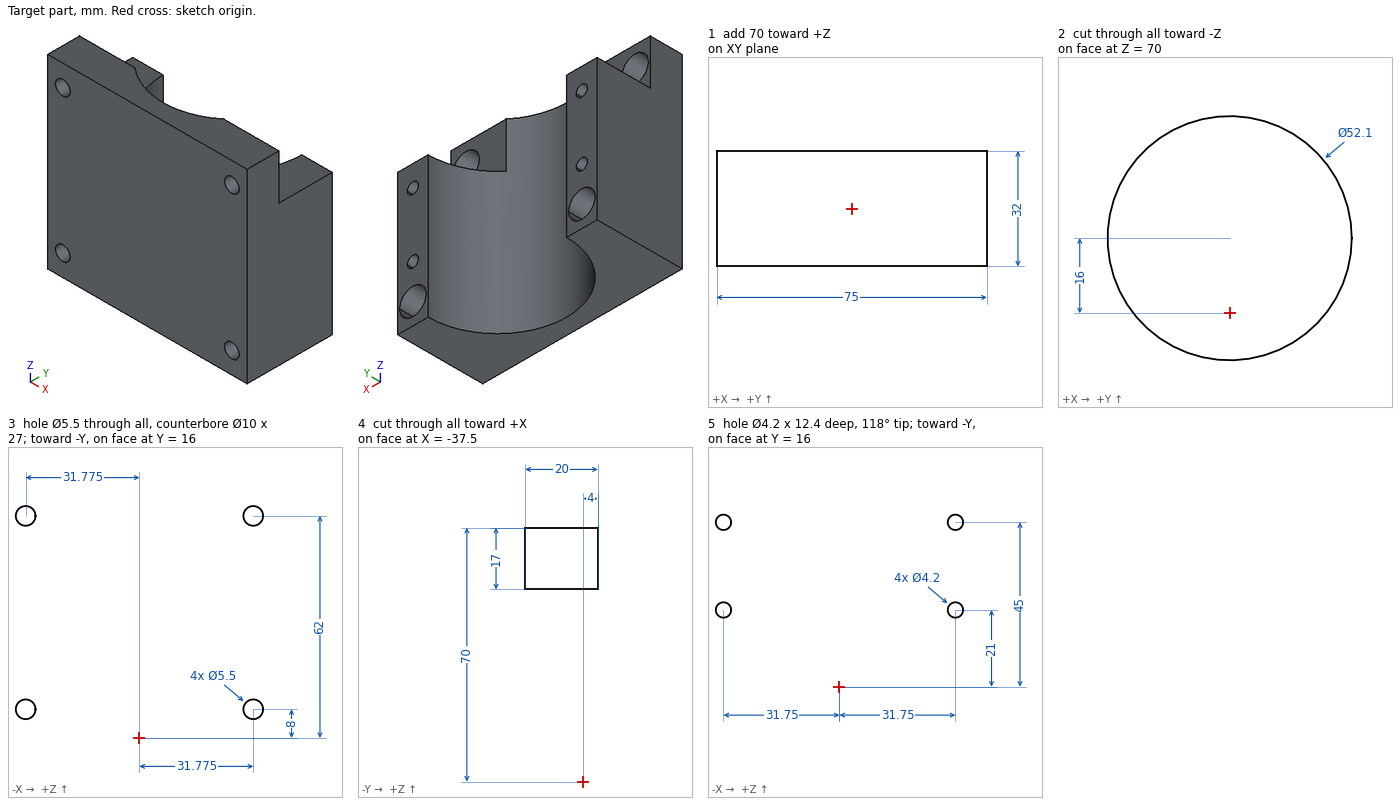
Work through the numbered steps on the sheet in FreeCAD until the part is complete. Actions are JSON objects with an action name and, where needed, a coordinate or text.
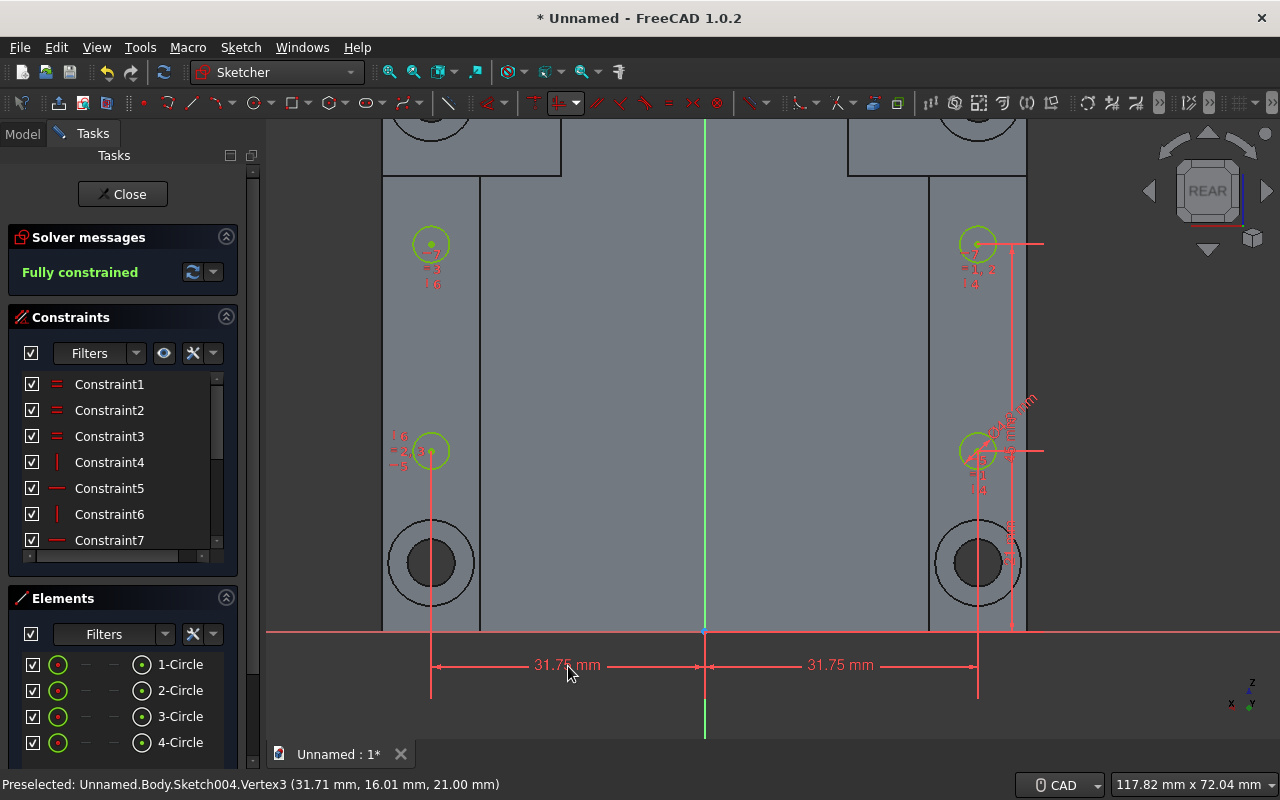
{"action": "left_click", "coordinate": [123, 194]}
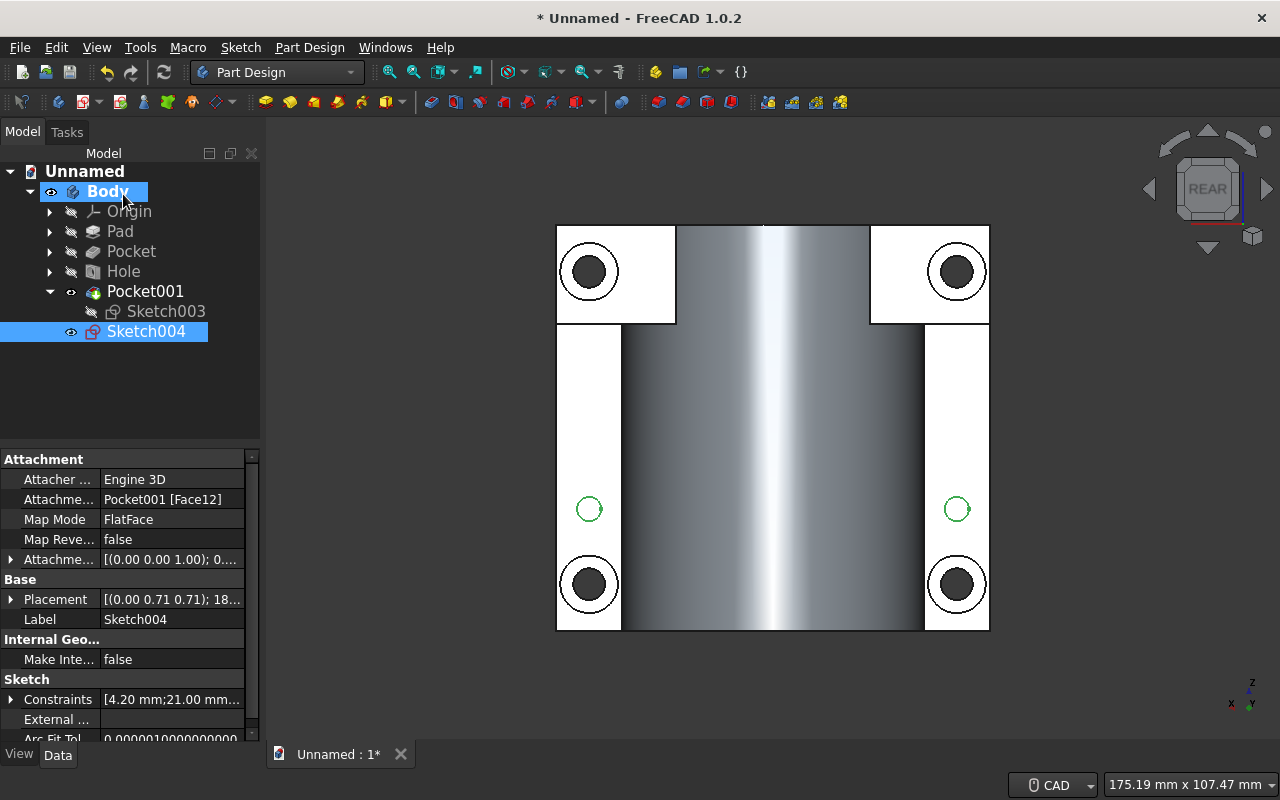
{"action": "left_click", "coordinate": [456, 102]}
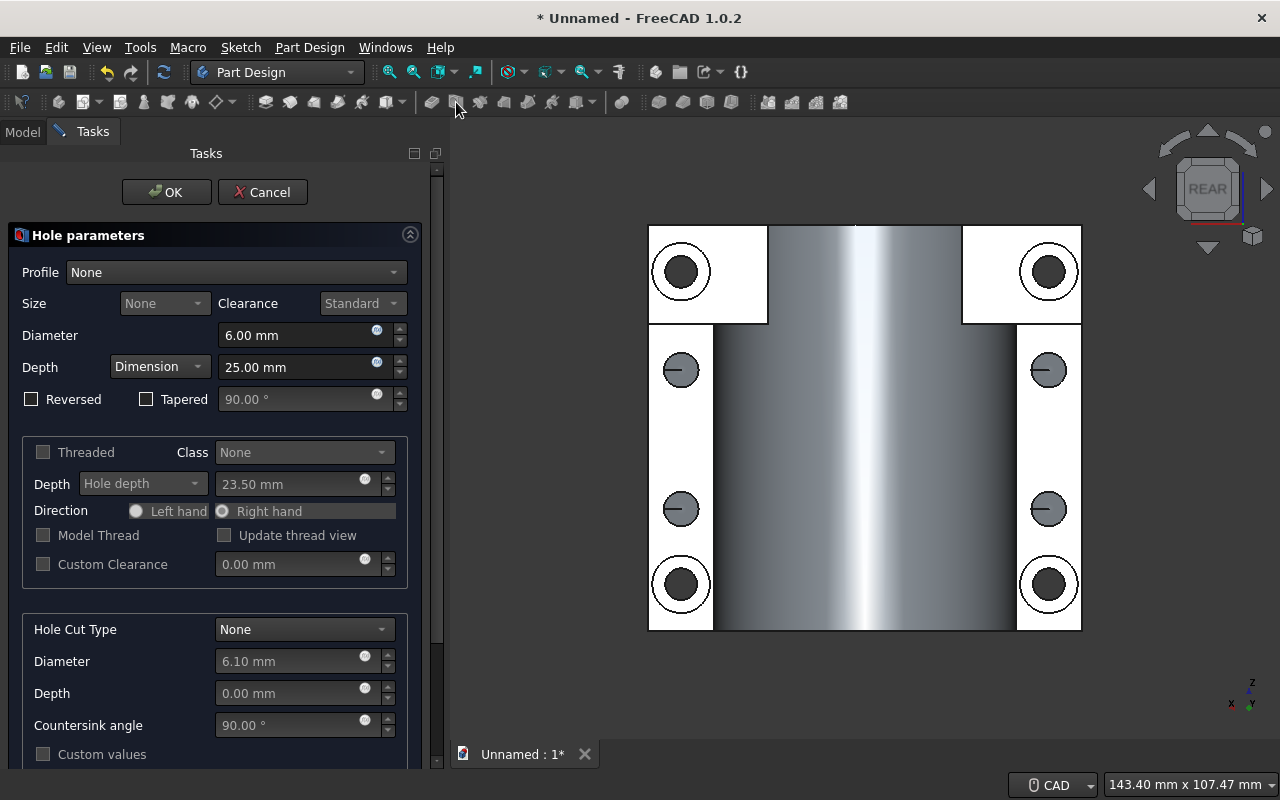
{"action": "triple_click", "coordinate": [305, 335]}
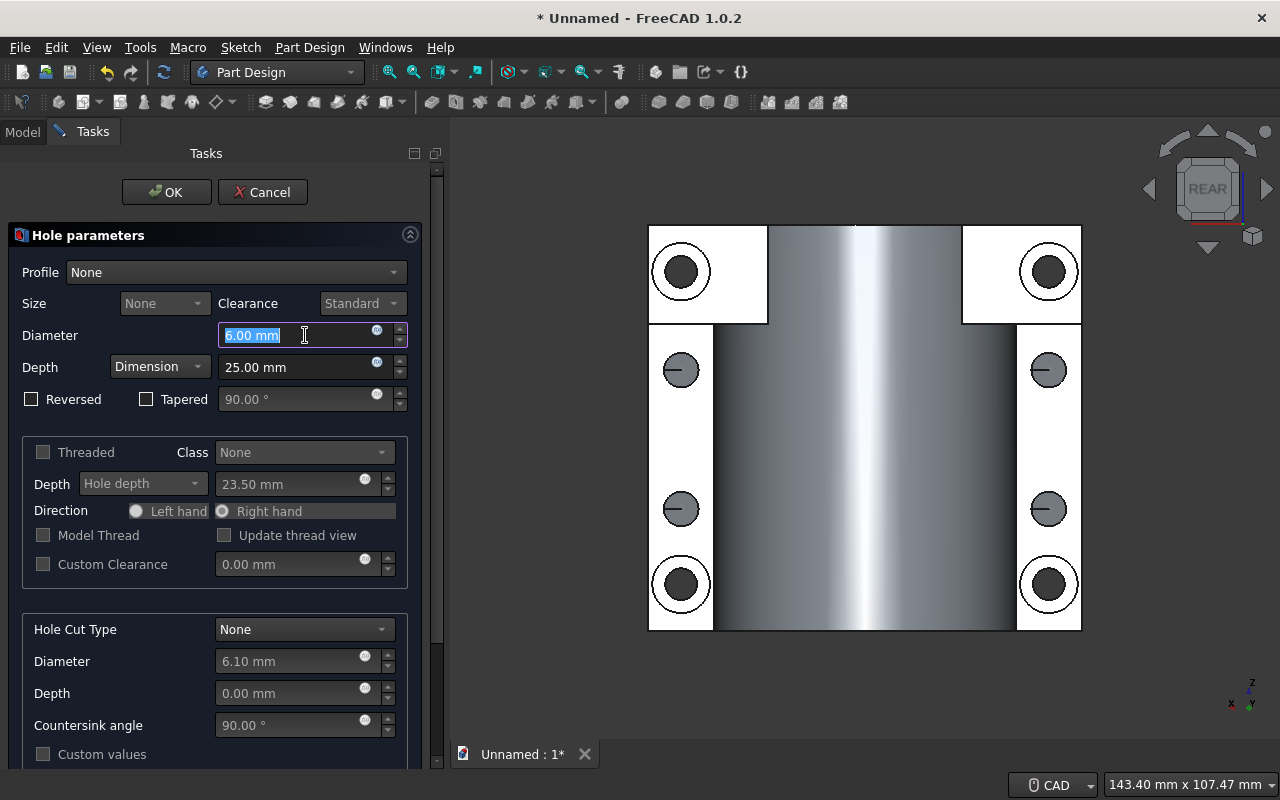
{"action": "type", "text": "4.2"}
{"action": "key", "text": "Tab"}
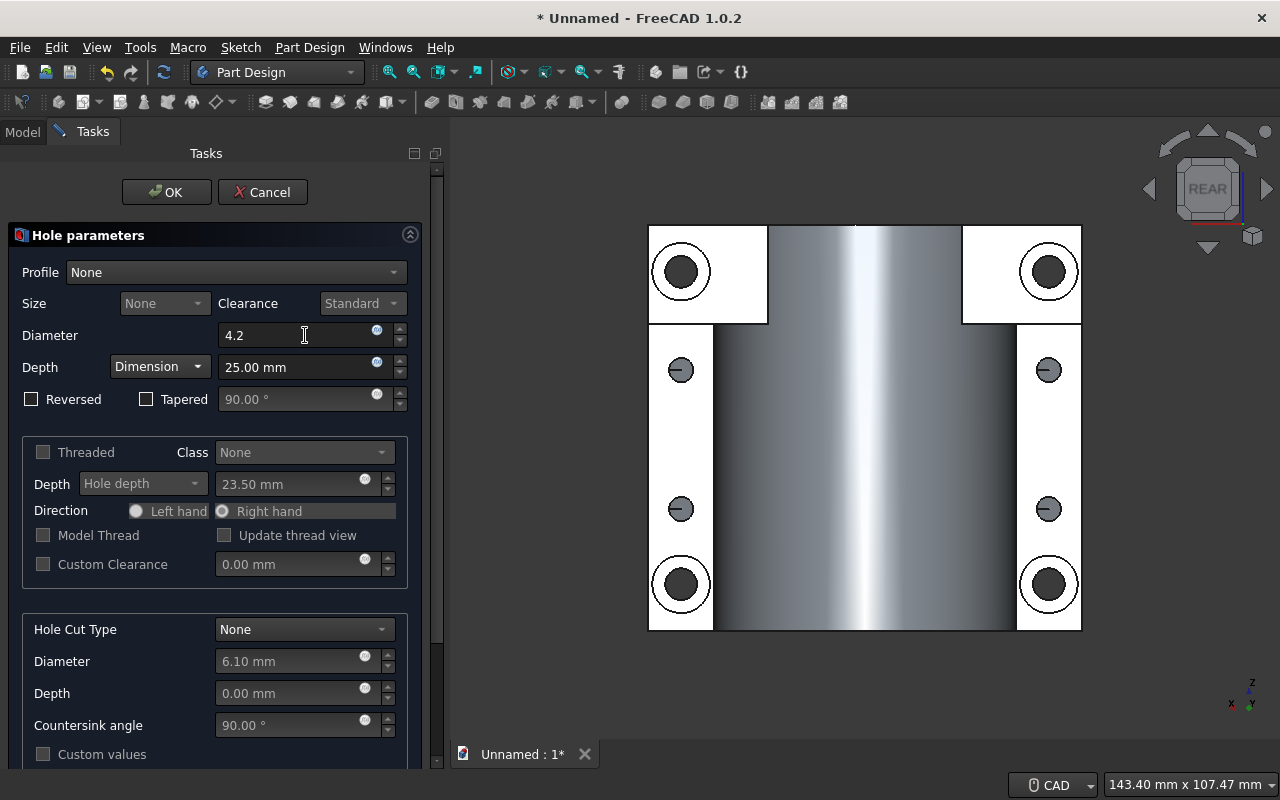
{"action": "triple_click", "coordinate": [305, 367]}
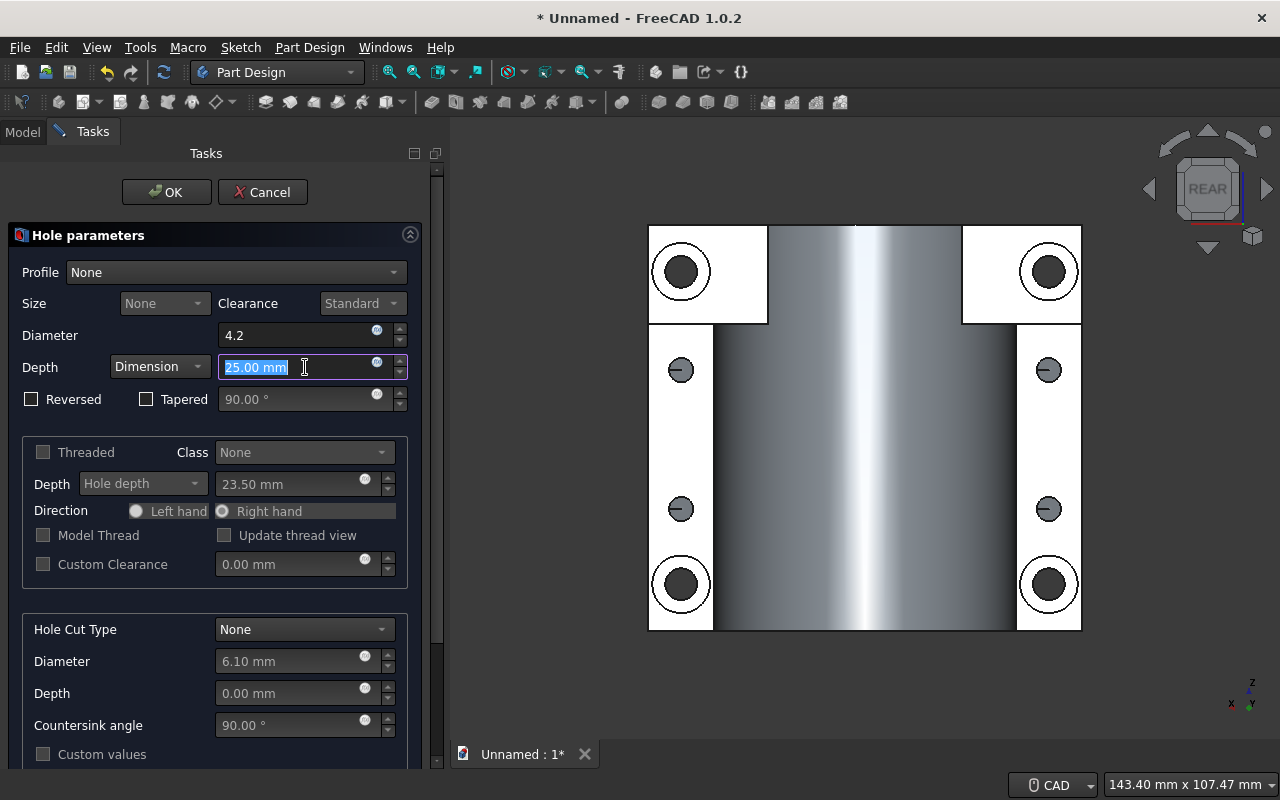
{"action": "type", "text": "12.4"}
{"action": "key", "text": "Tab"}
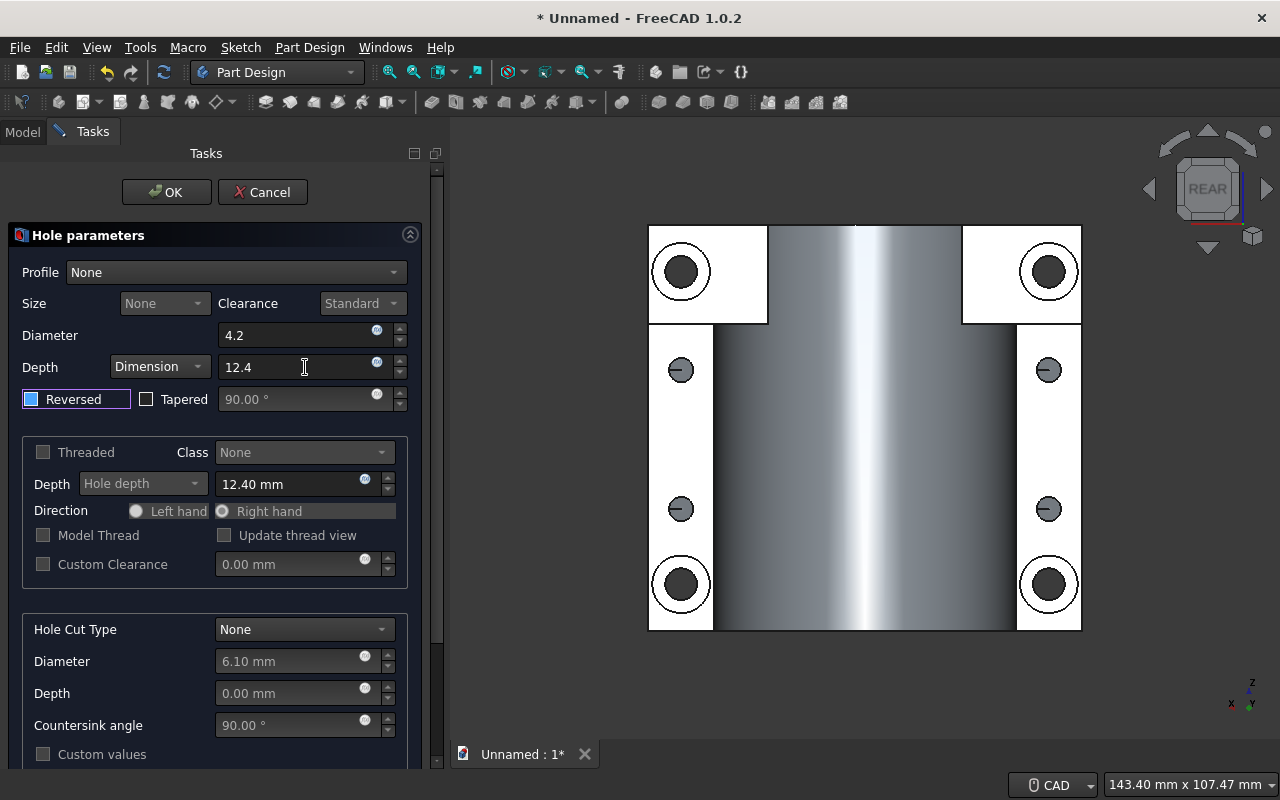
{"action": "left_click", "coordinate": [167, 192]}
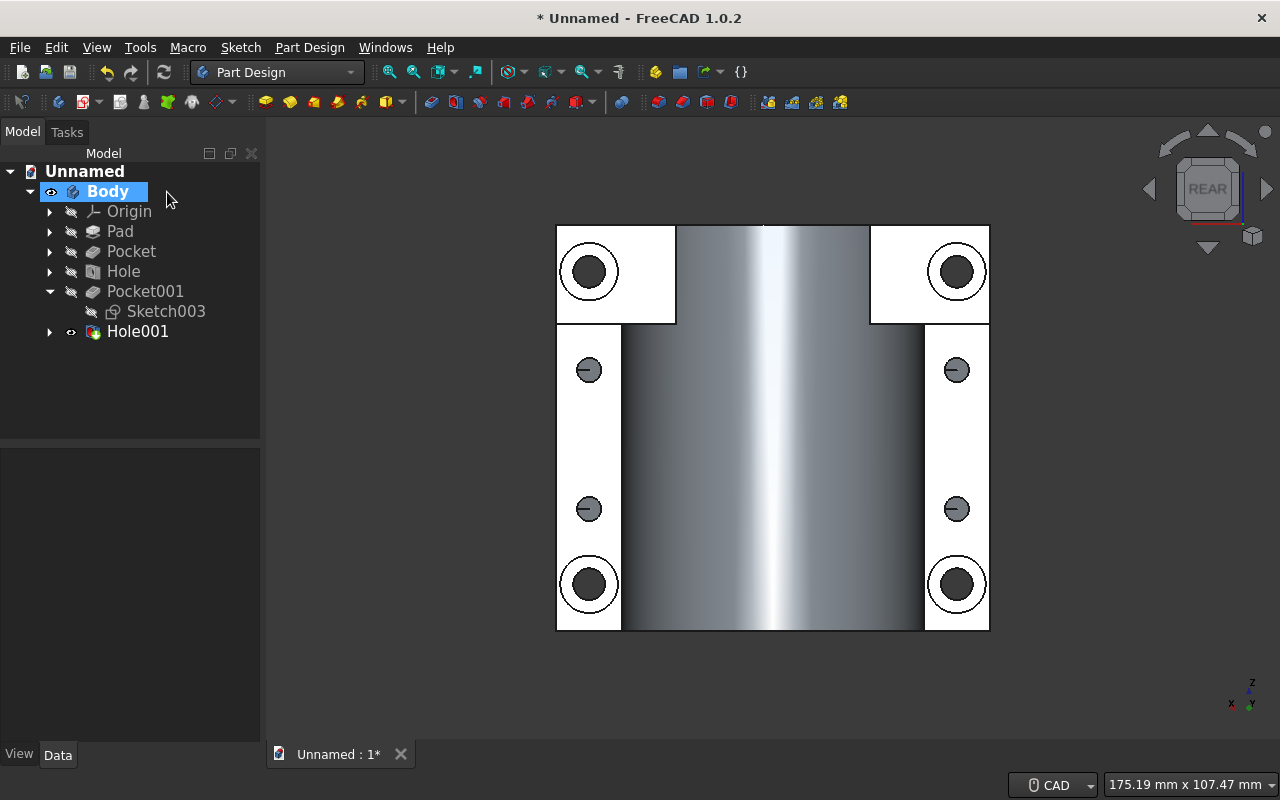
{"action": "key", "text": "0"}